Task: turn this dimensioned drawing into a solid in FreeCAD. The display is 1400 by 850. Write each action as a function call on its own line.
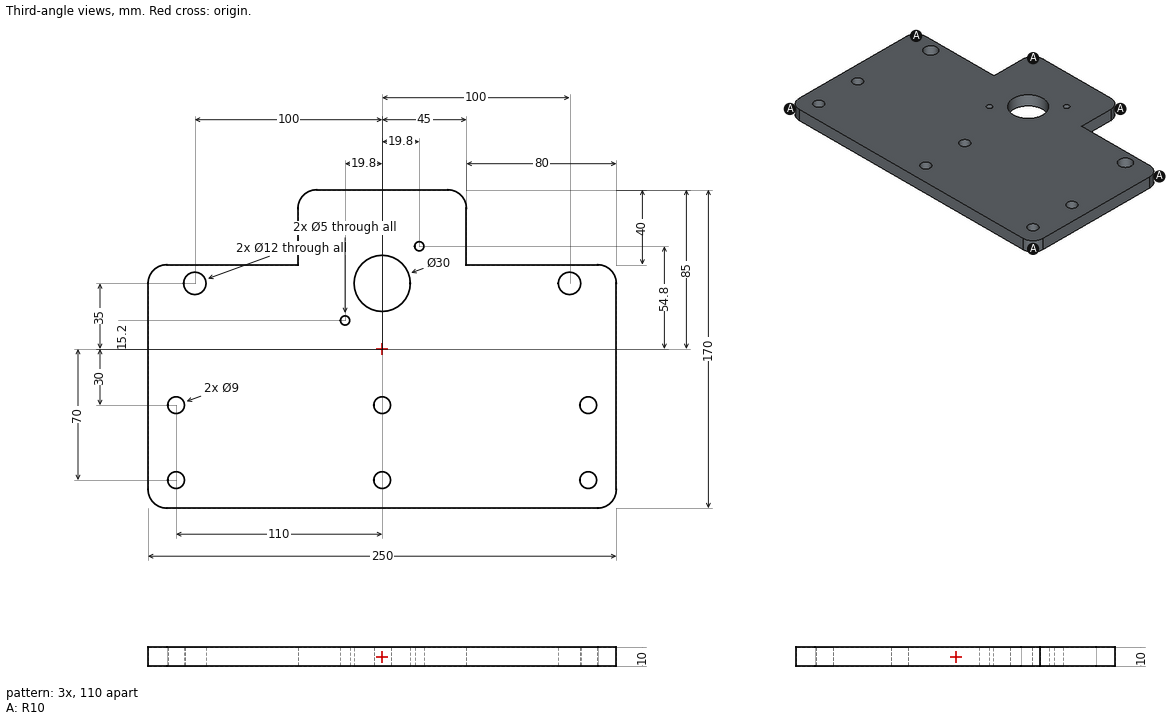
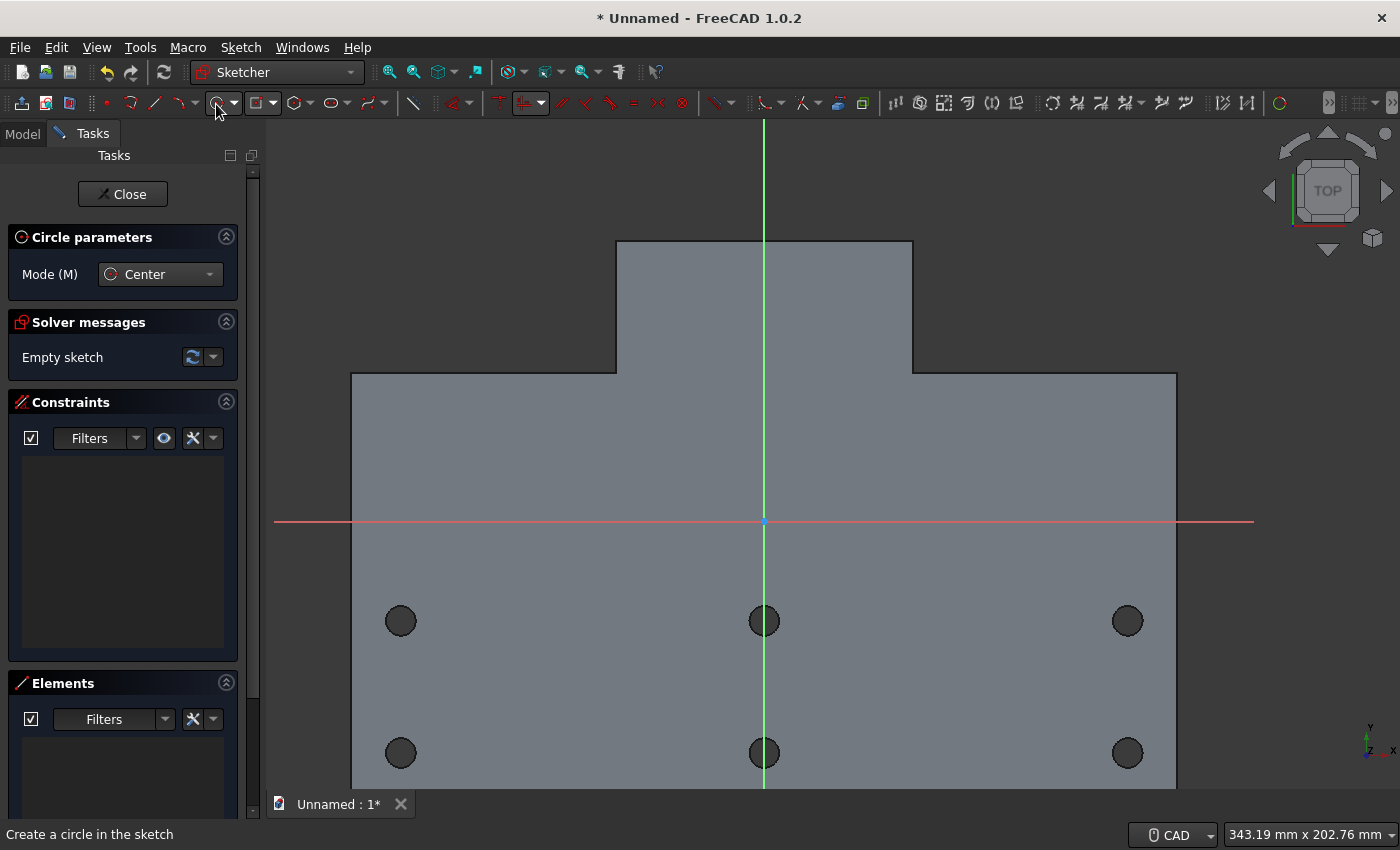
click(434, 406)
move(448, 392)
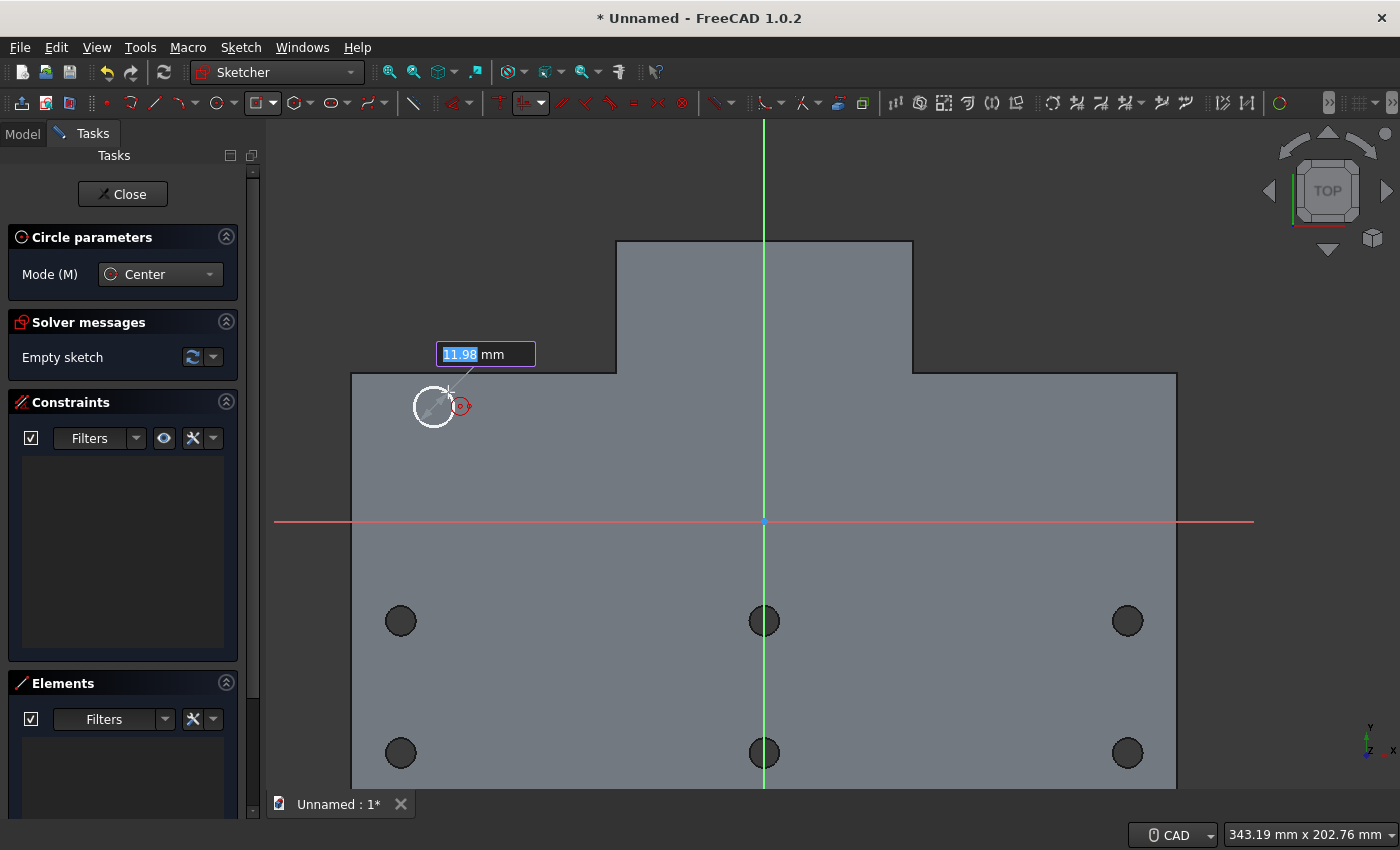
text(12)
key(Return)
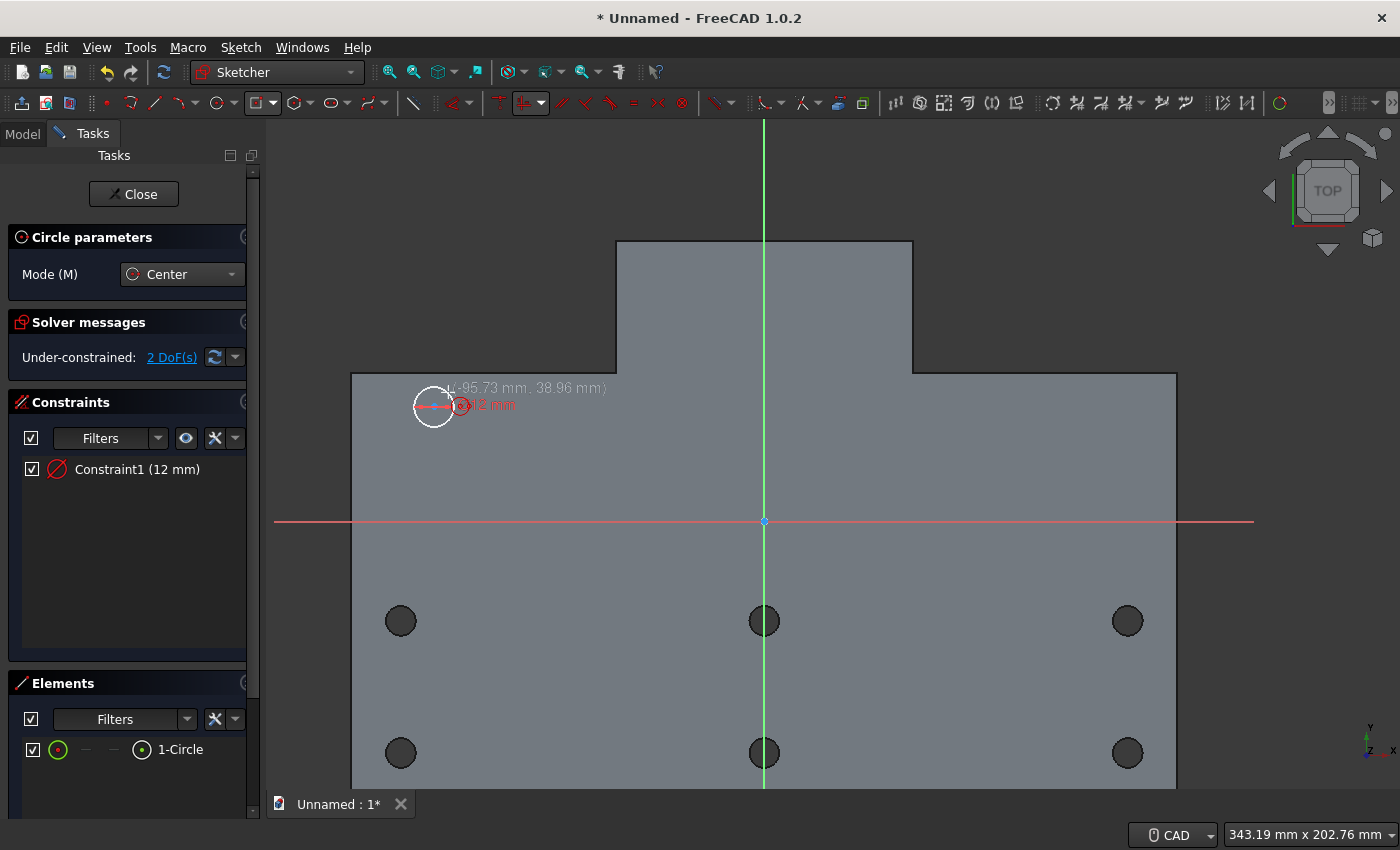
click(1095, 406)
move(1109, 392)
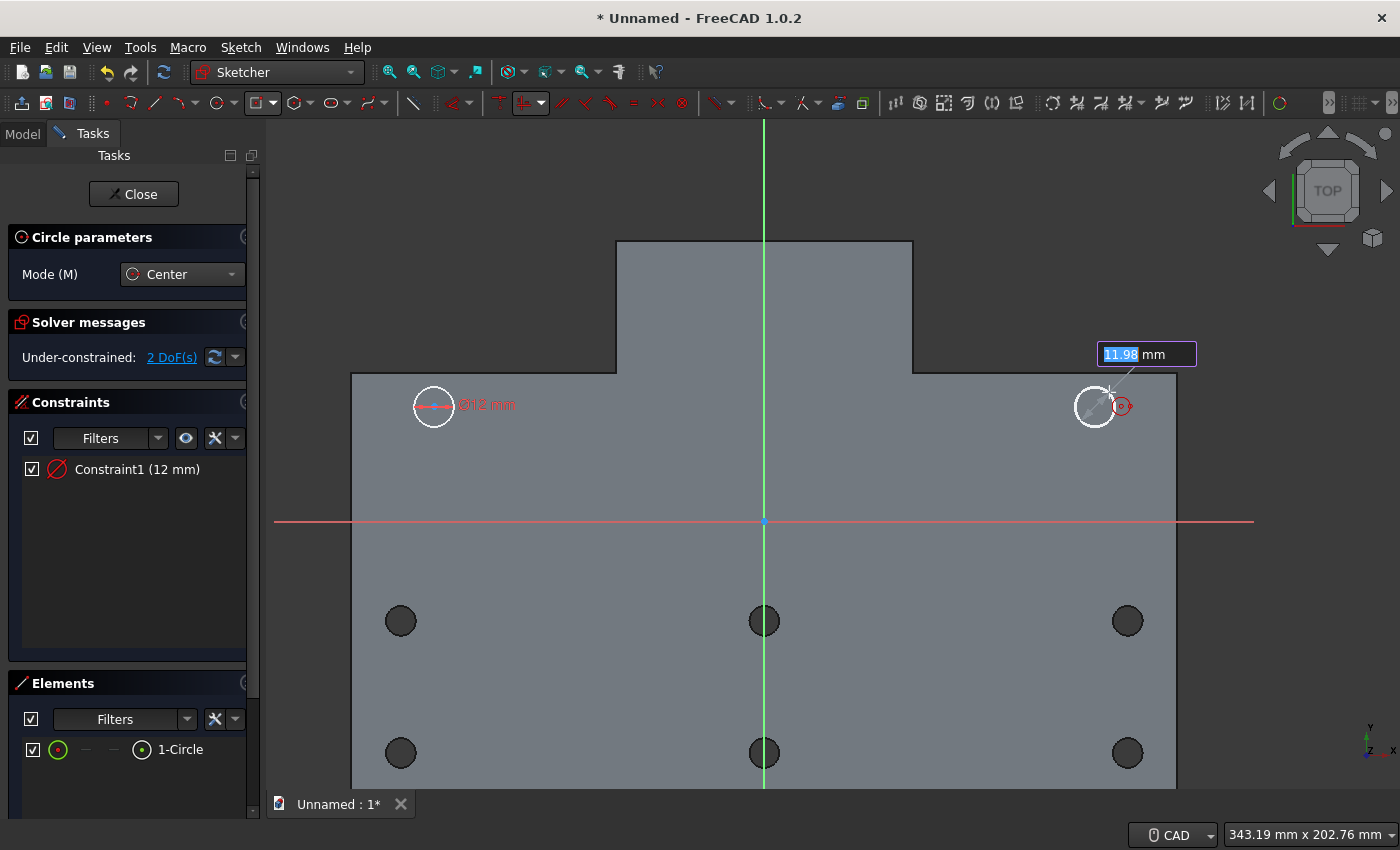
text(12)
key(Return)
key(Escape)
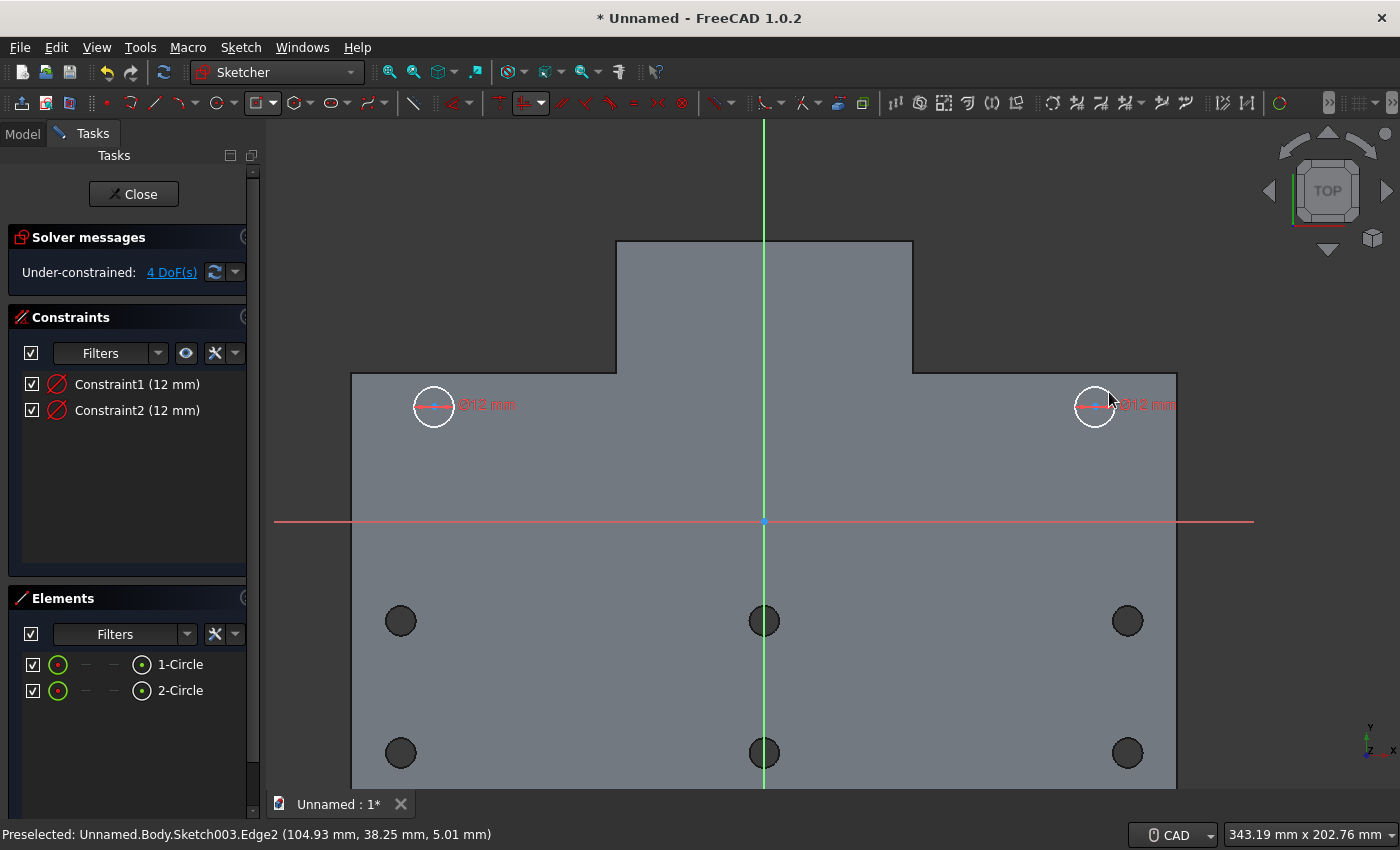
click(434, 407)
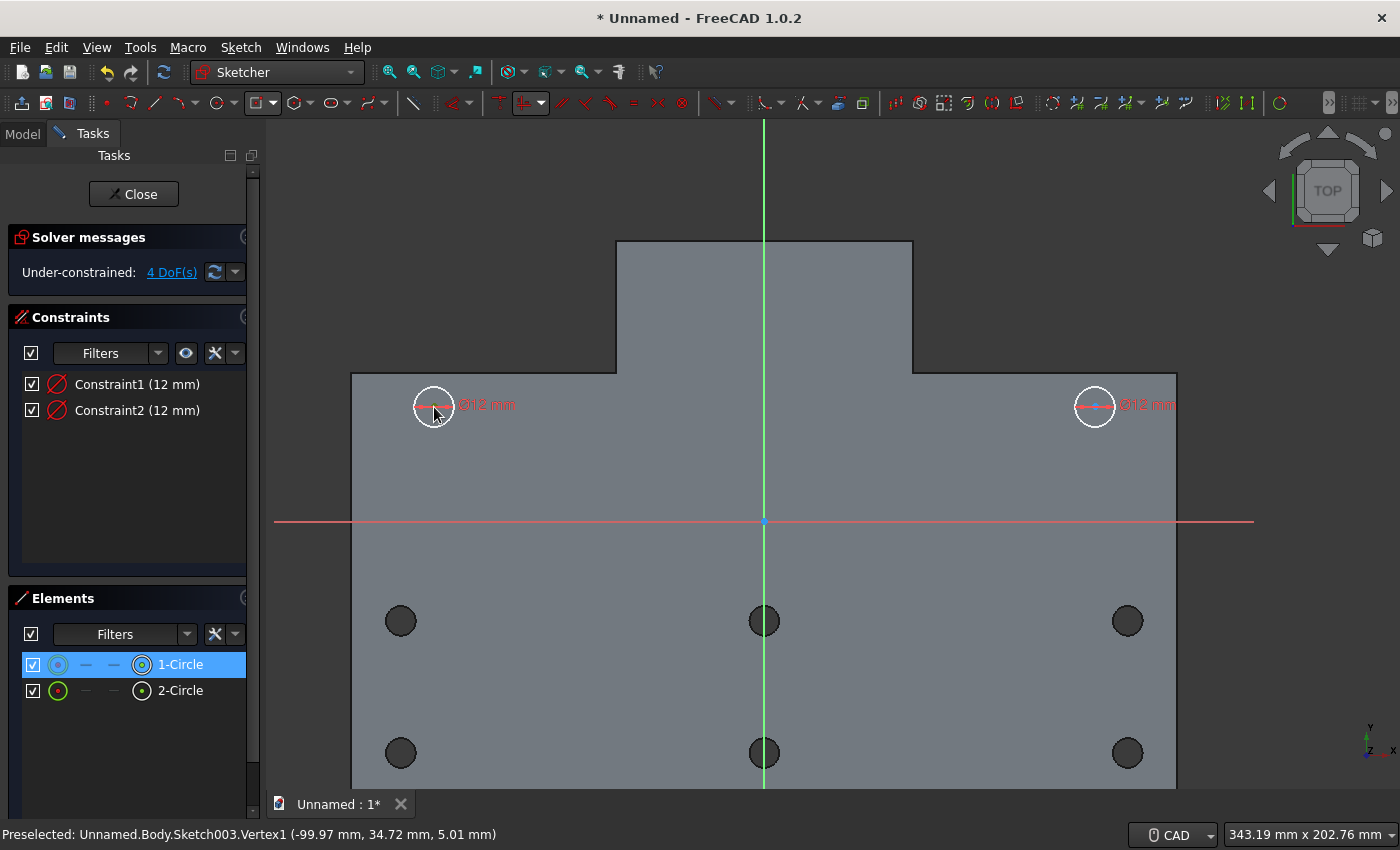
click(1095, 407)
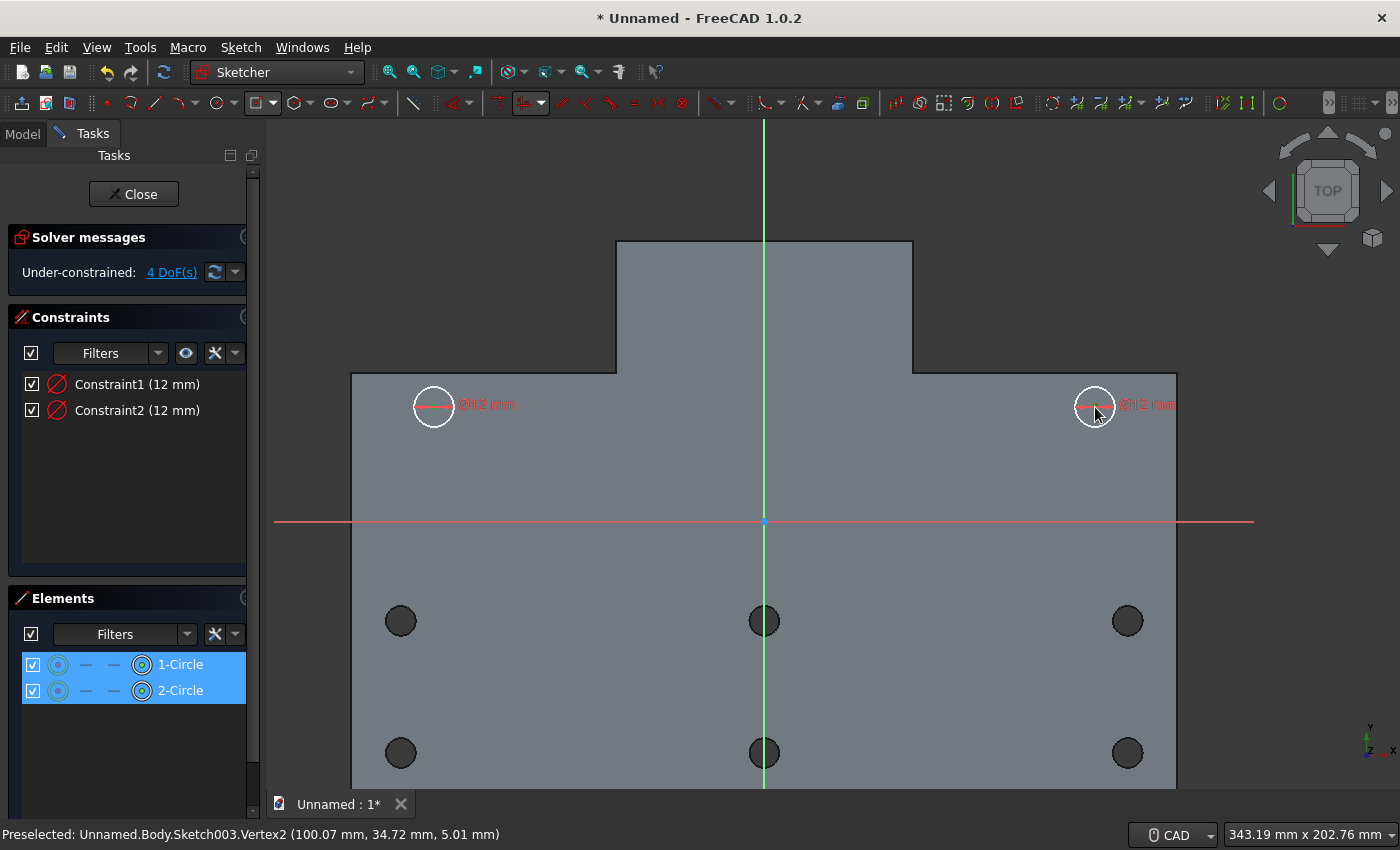
click(544, 104)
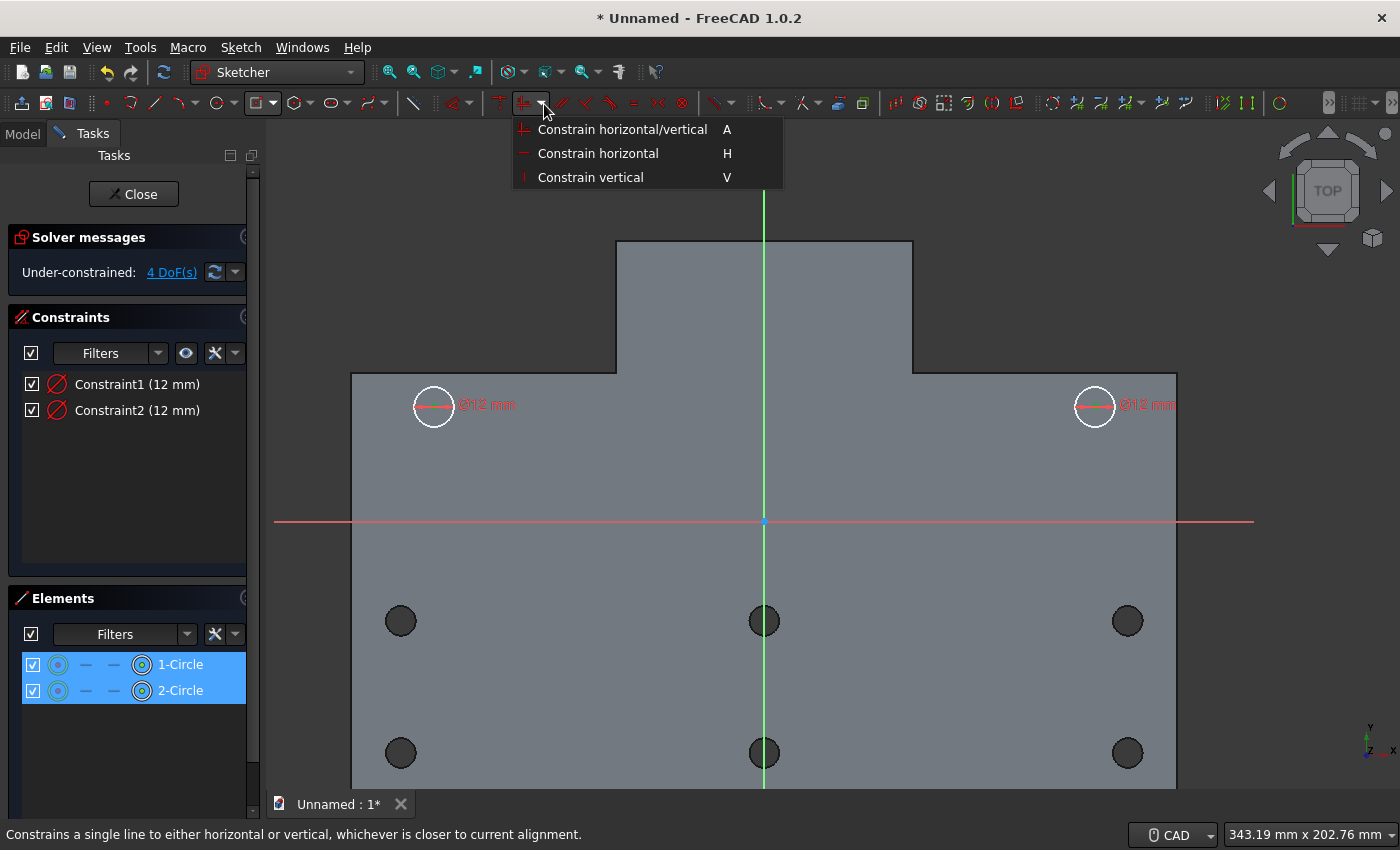
click(648, 153)